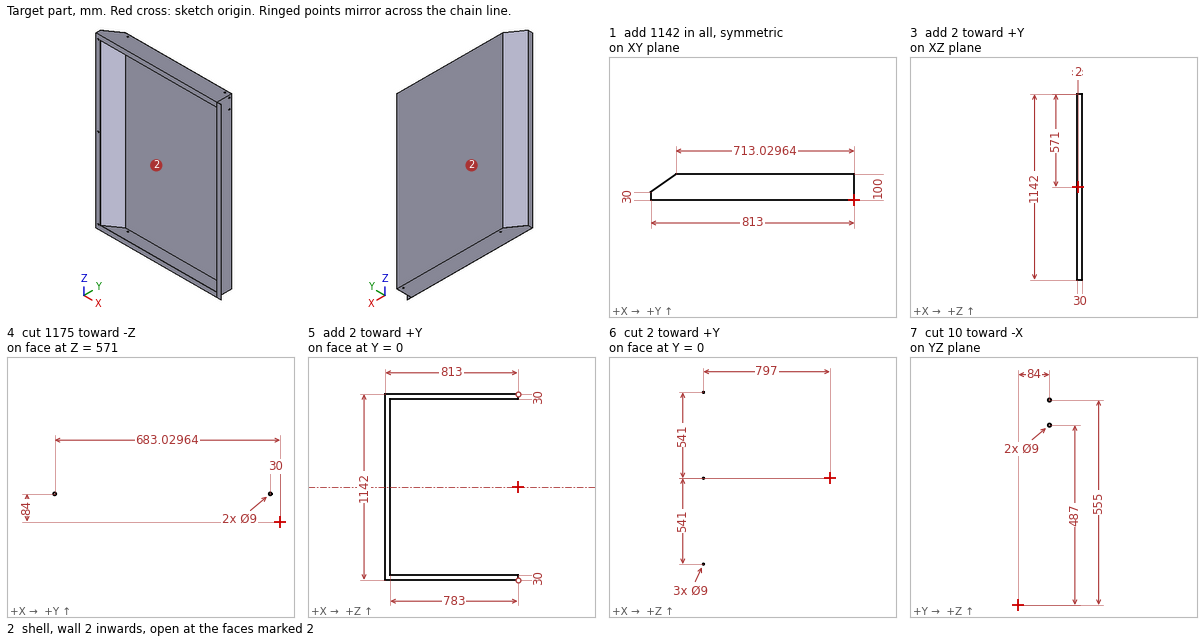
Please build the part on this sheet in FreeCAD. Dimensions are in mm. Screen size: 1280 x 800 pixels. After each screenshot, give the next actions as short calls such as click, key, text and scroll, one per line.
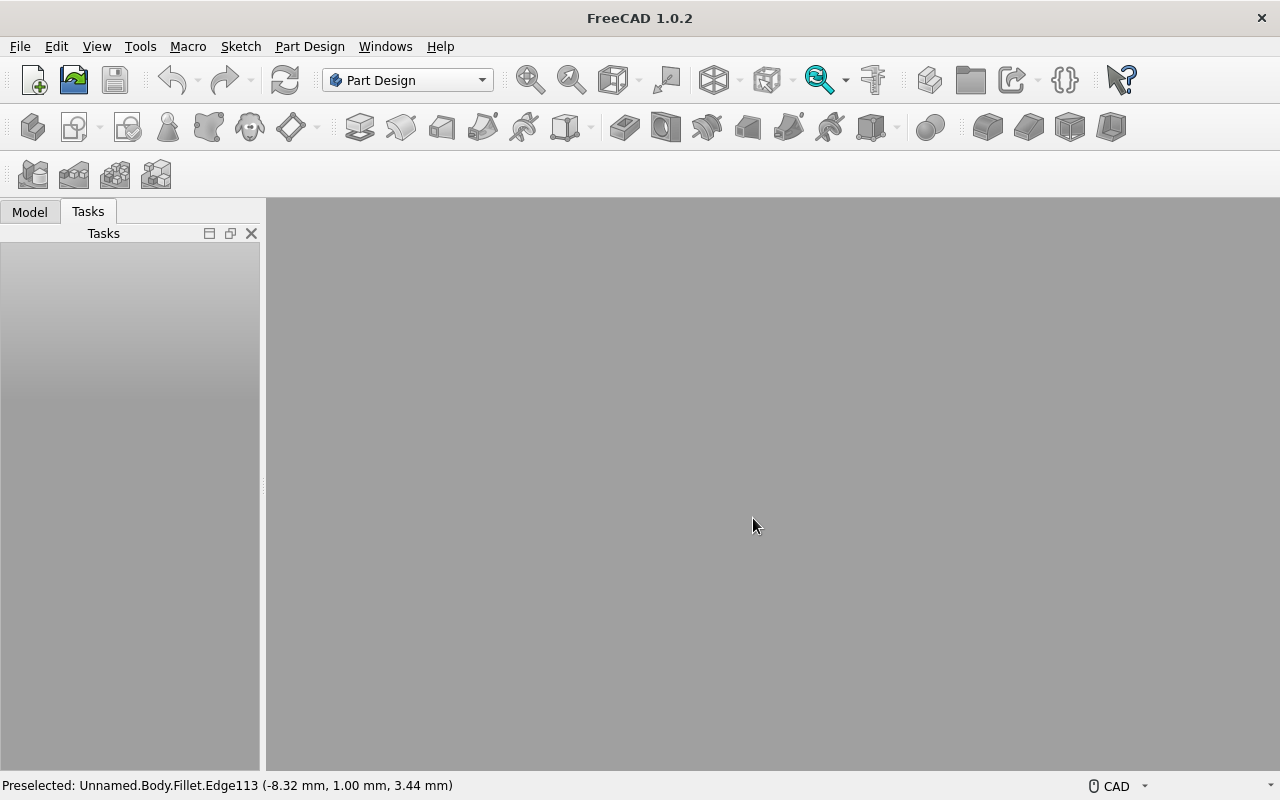
click(33, 80)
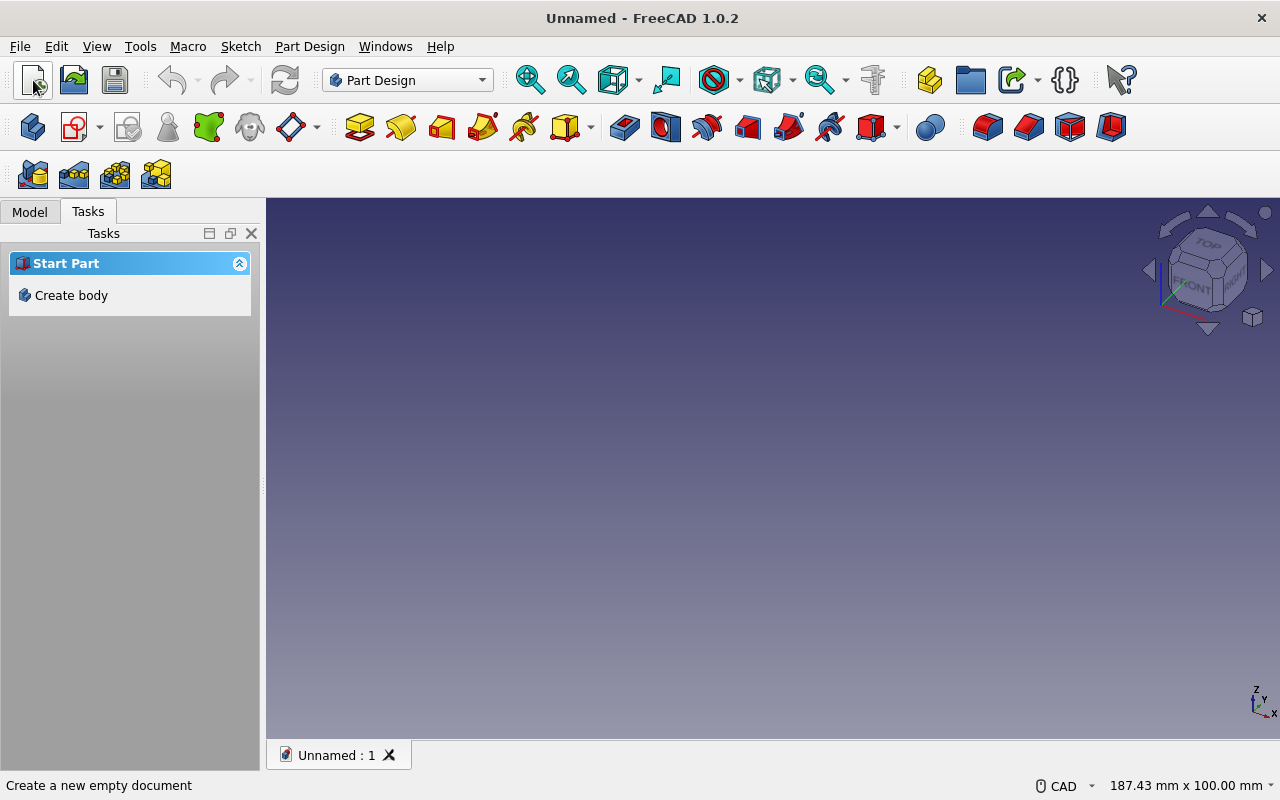
click(74, 128)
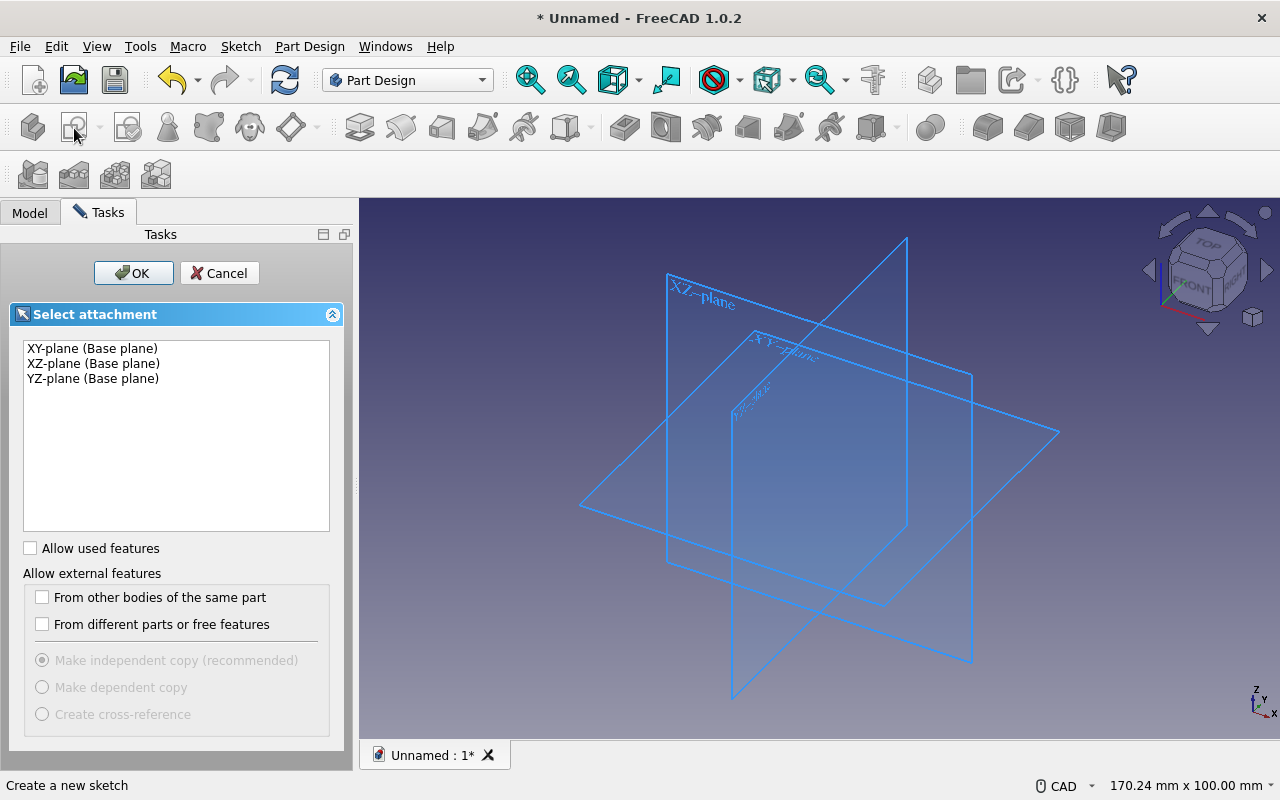
click(84, 348)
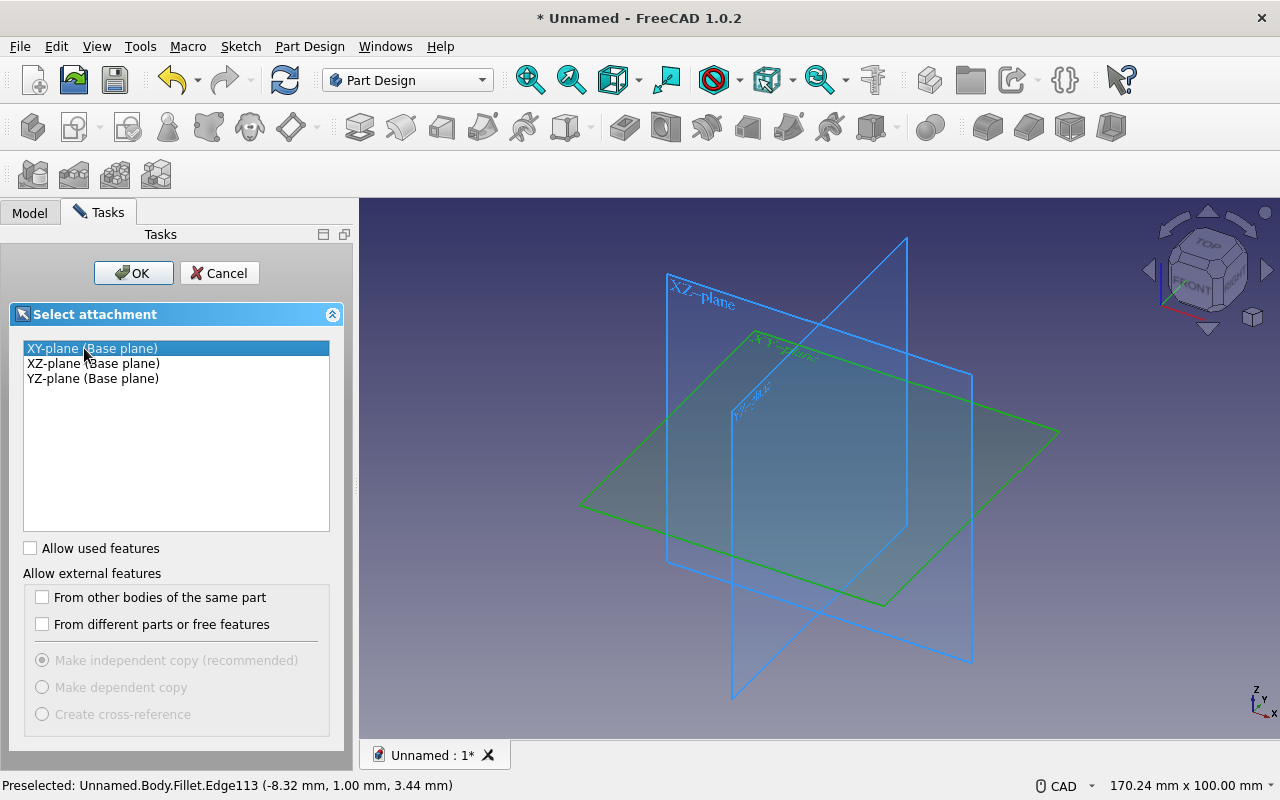
click(134, 273)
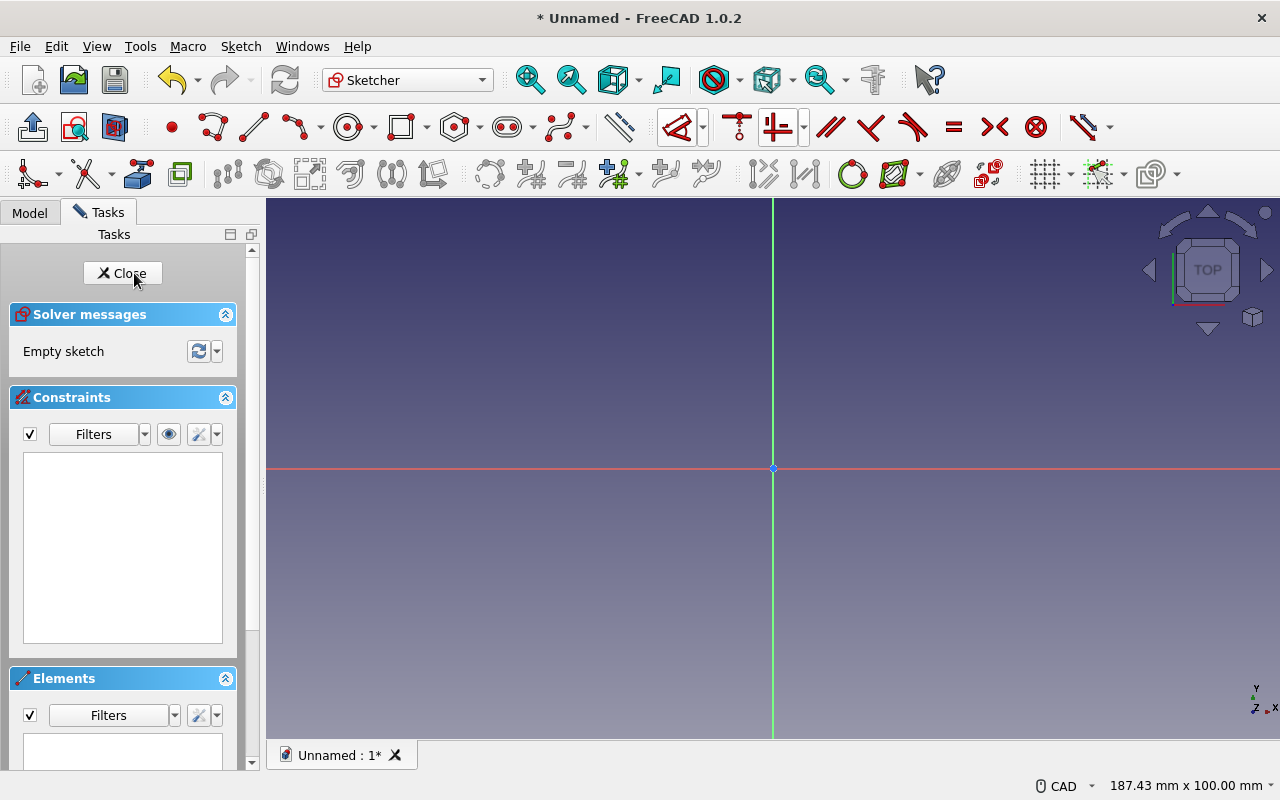
scroll(1038, 511, down, 10)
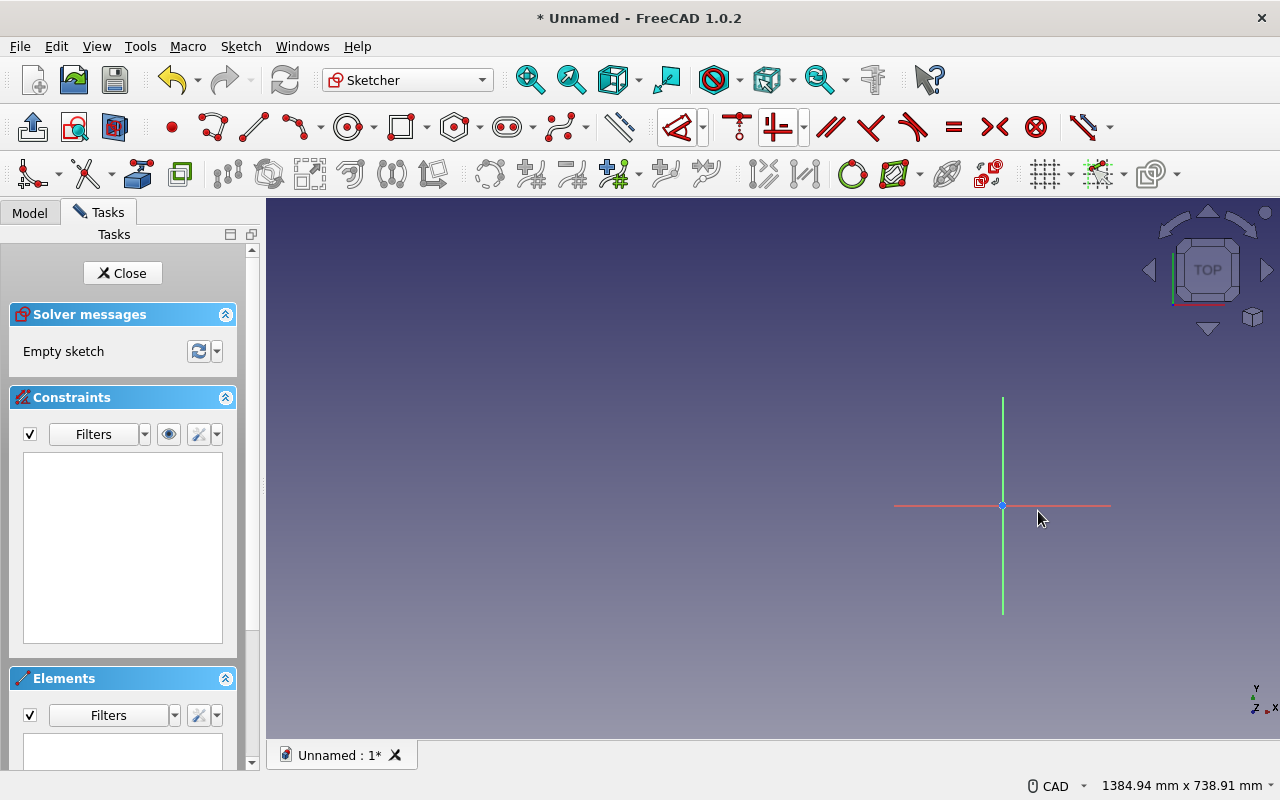
click(213, 128)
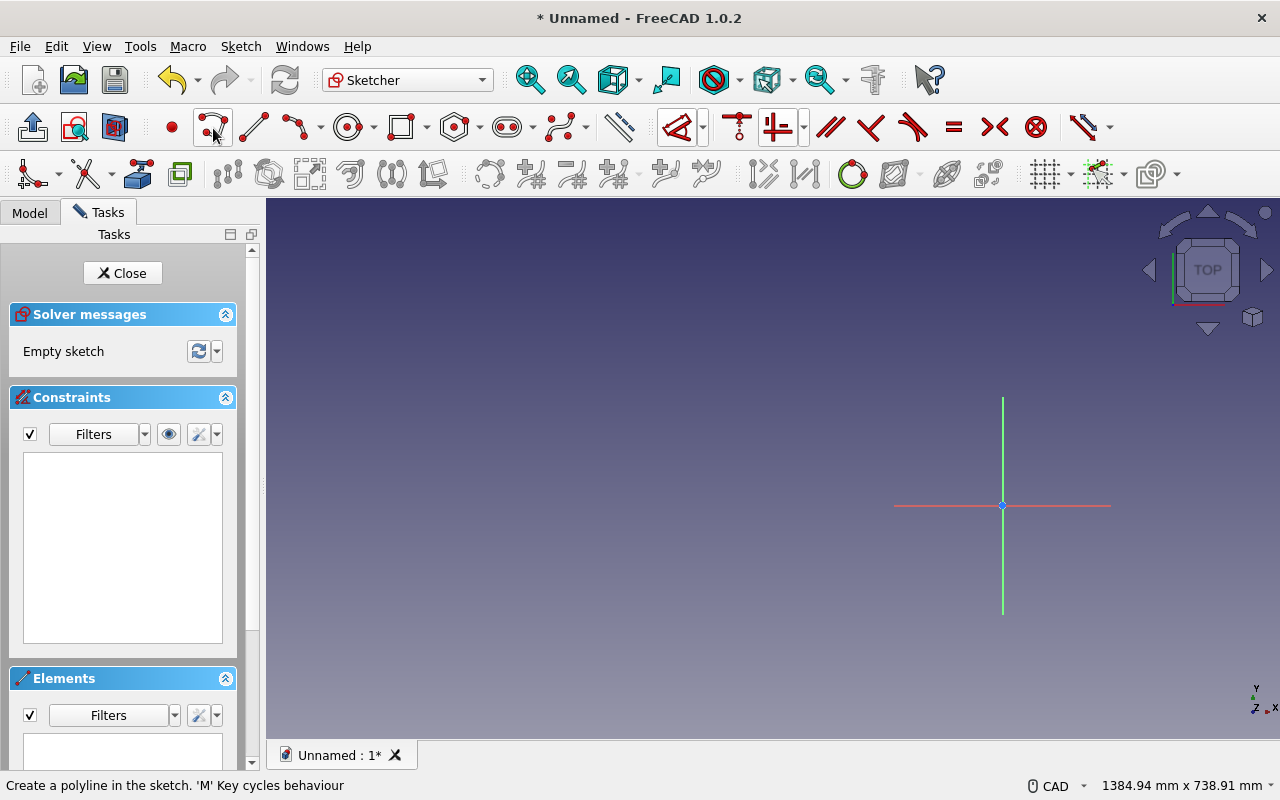
click(1003, 506)
click(994, 433)
click(481, 433)
click(408, 484)
click(408, 497)
click(1003, 506)
key(Escape)
key(Escape)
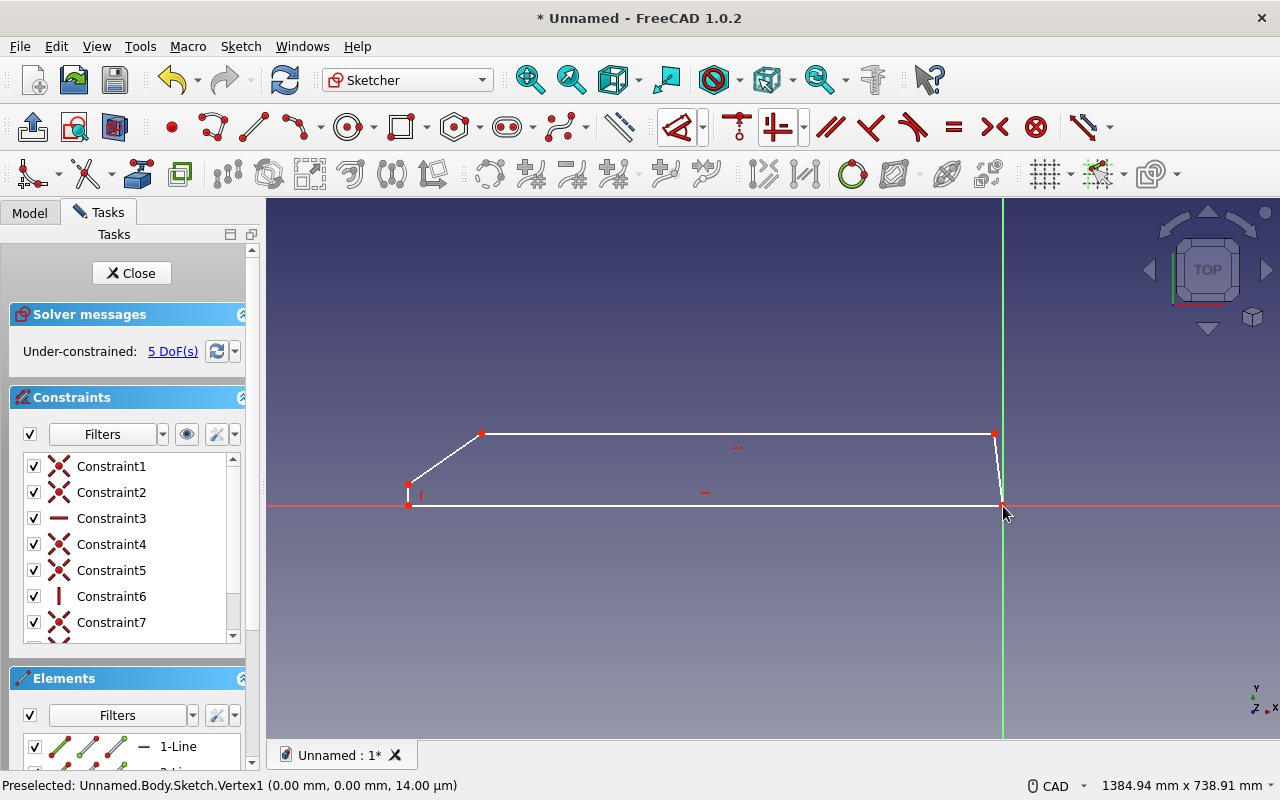
click(1000, 484)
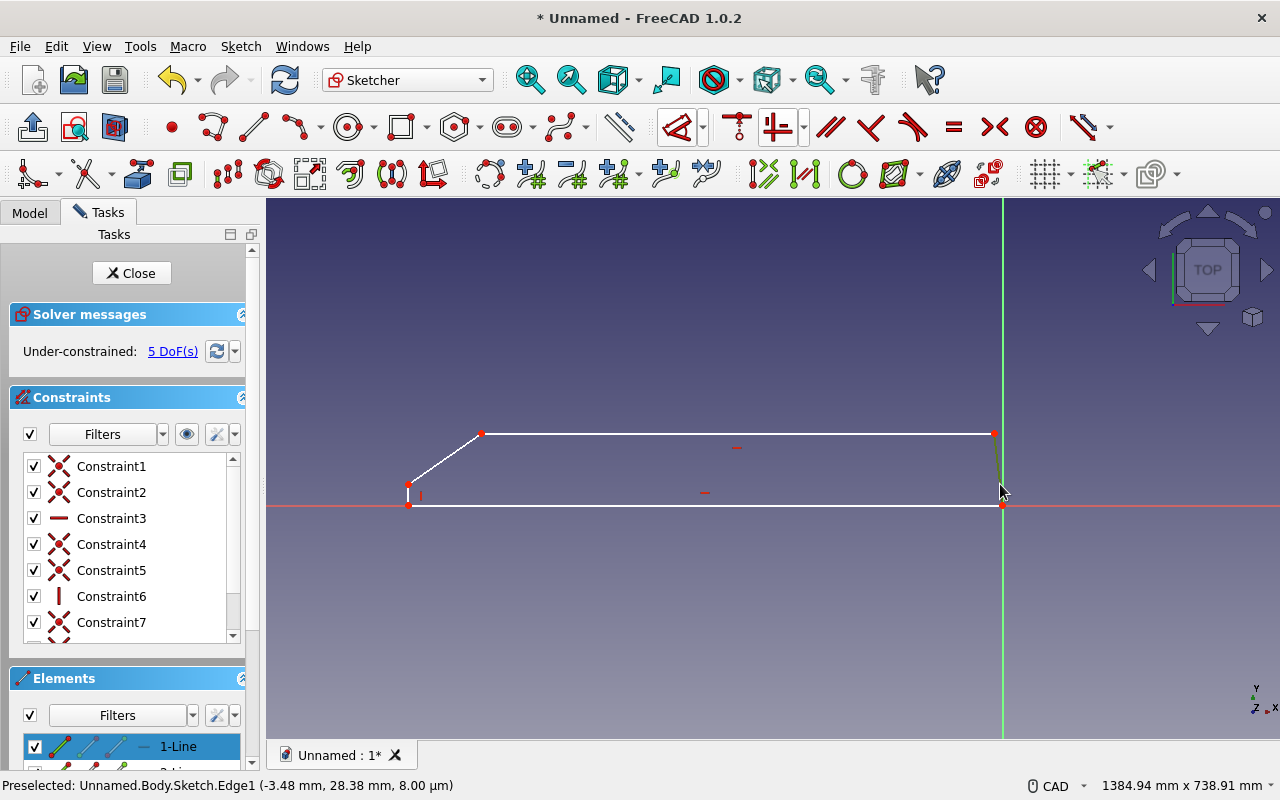
click(804, 128)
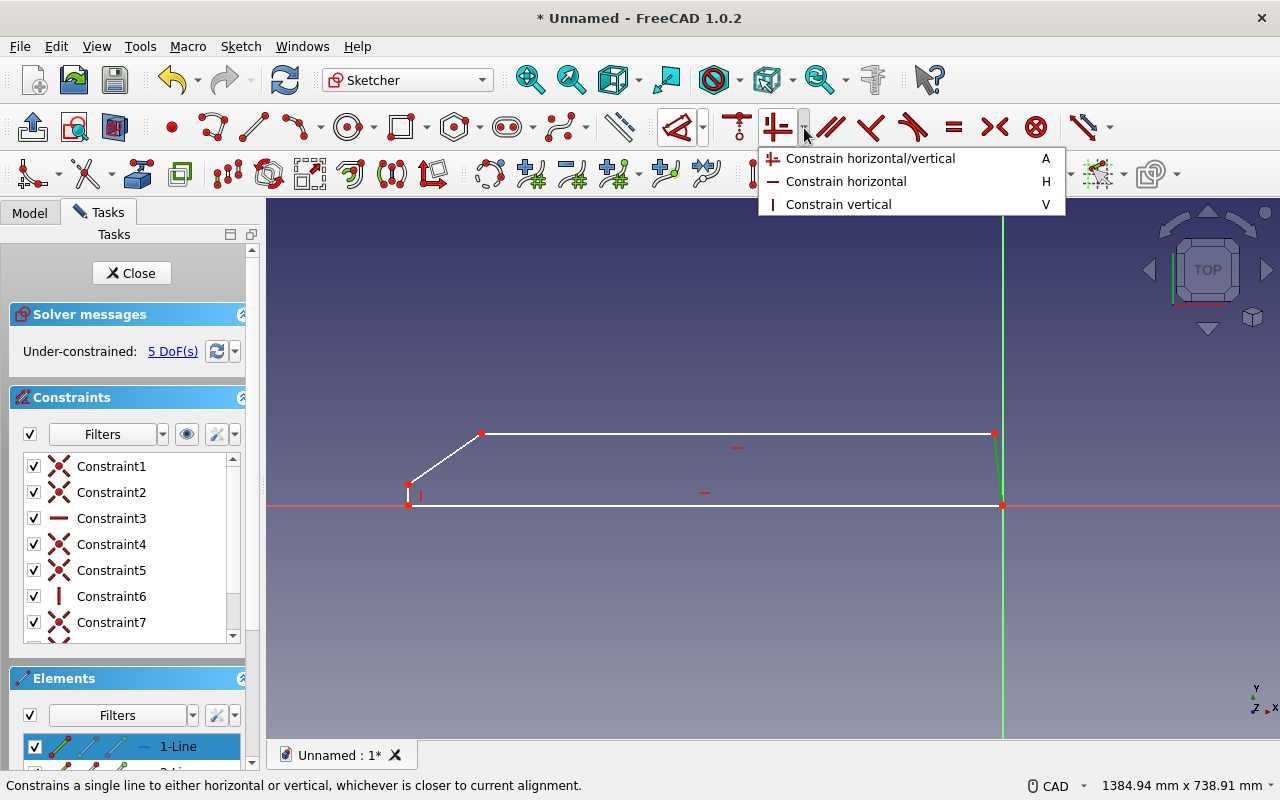
click(912, 204)